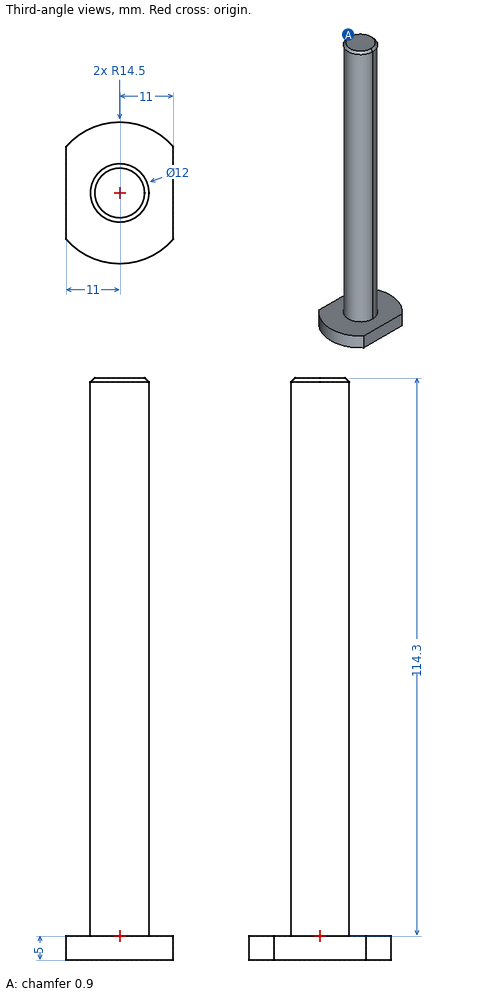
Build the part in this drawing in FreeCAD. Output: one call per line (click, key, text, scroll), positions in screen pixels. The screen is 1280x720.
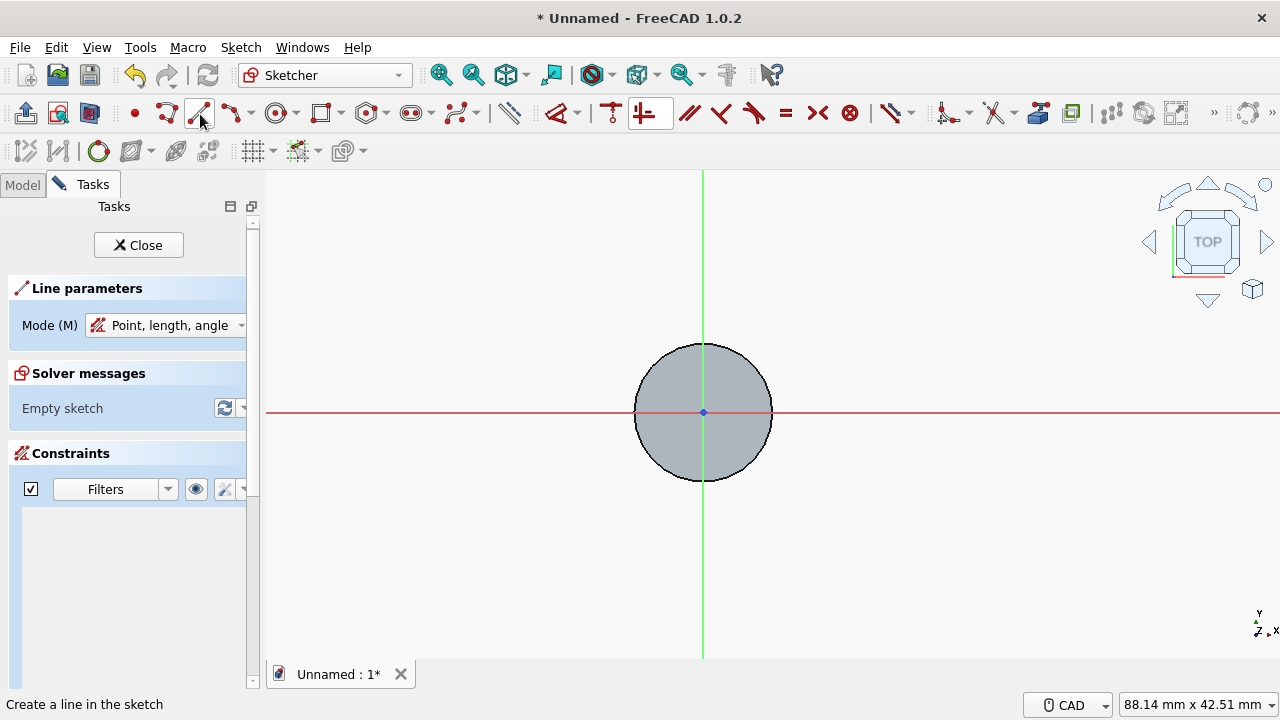
click(577, 521)
click(577, 304)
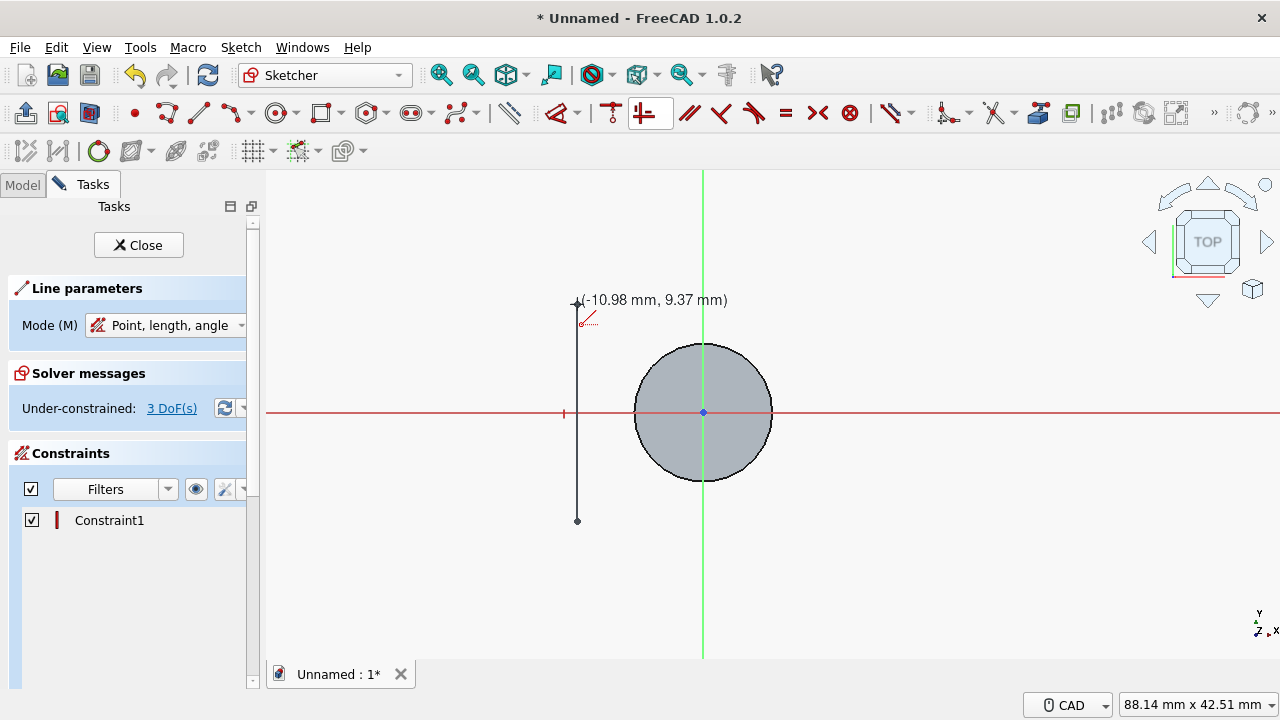
click(830, 304)
click(830, 521)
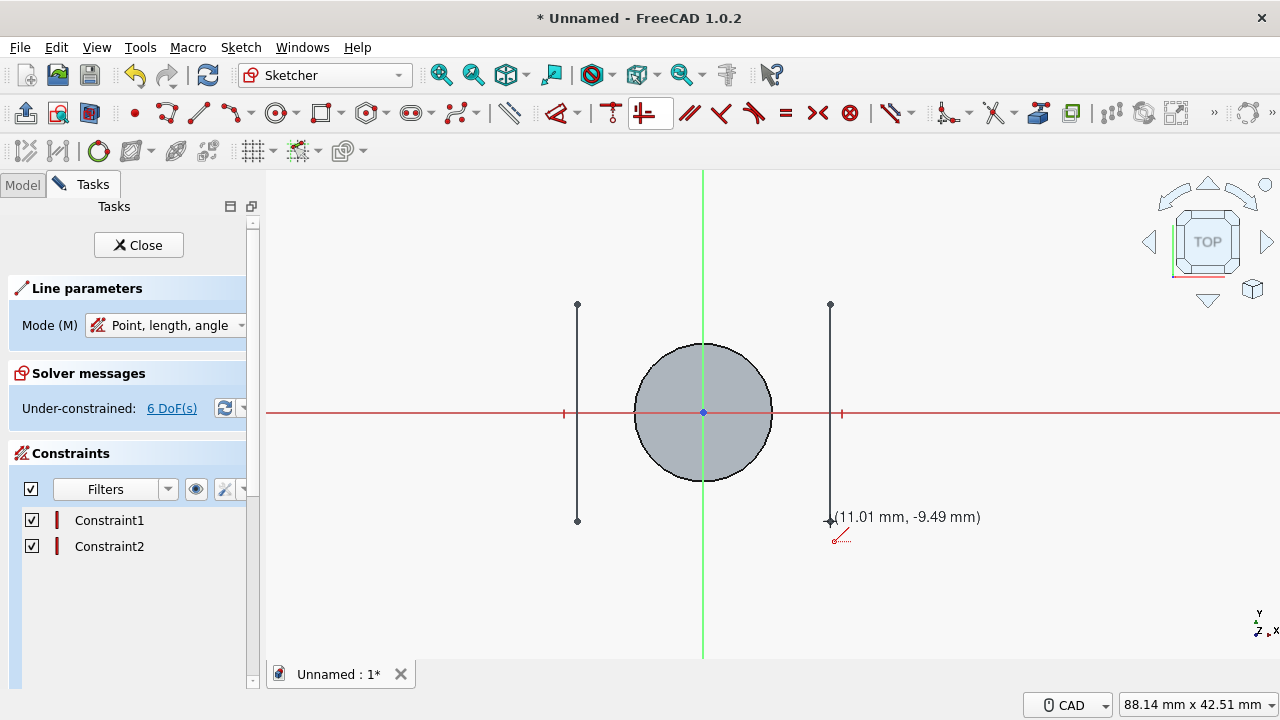
click(232, 114)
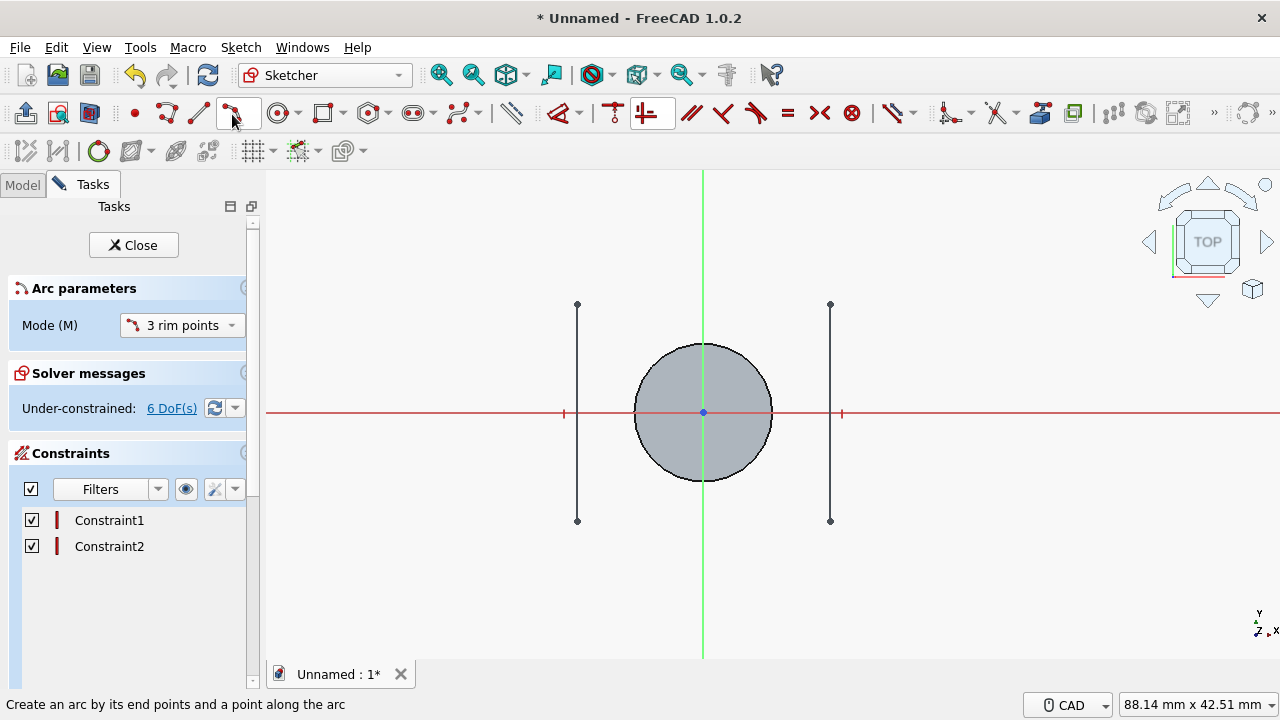
click(577, 305)
click(830, 305)
click(732, 248)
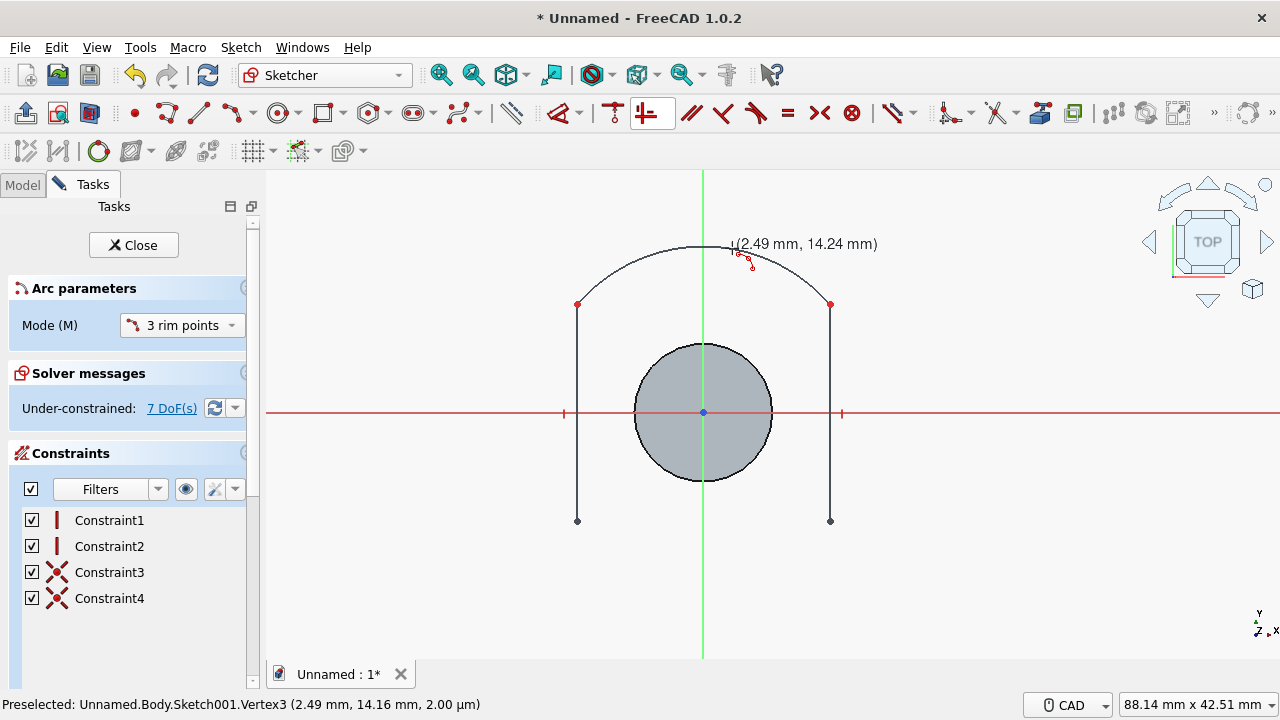
click(830, 522)
click(577, 522)
click(675, 577)
key(Escape)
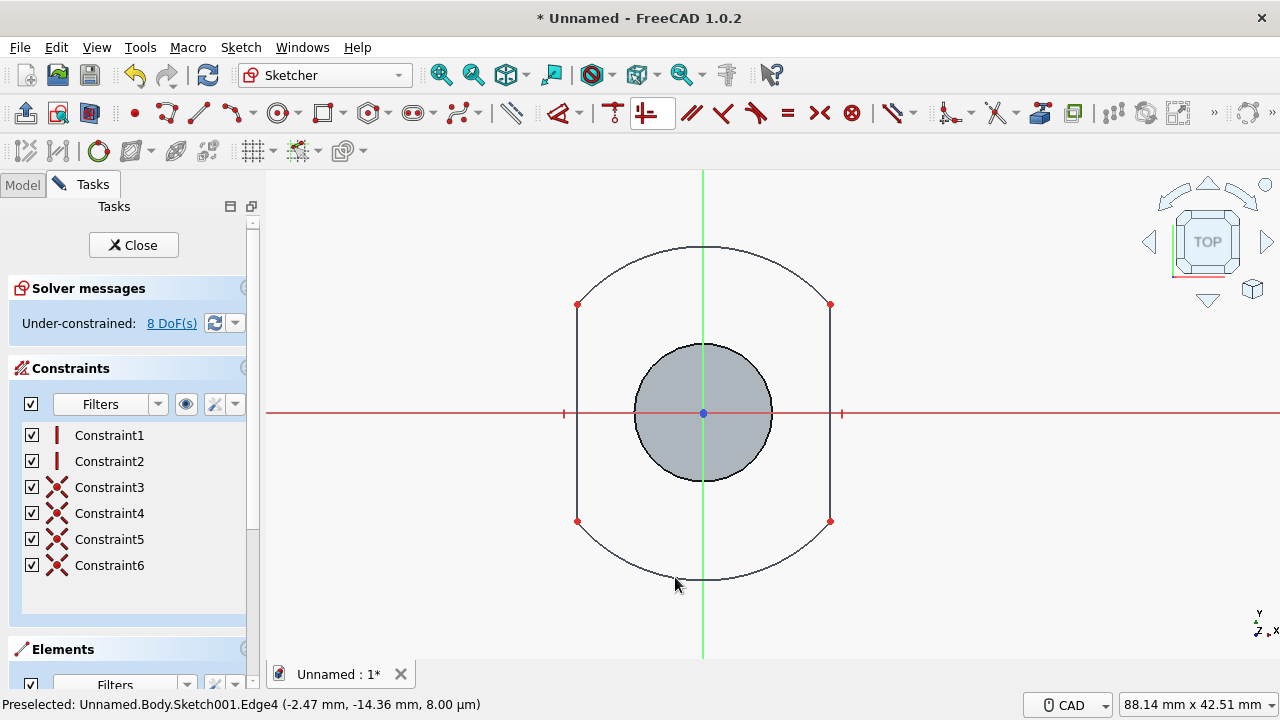
click(760, 256)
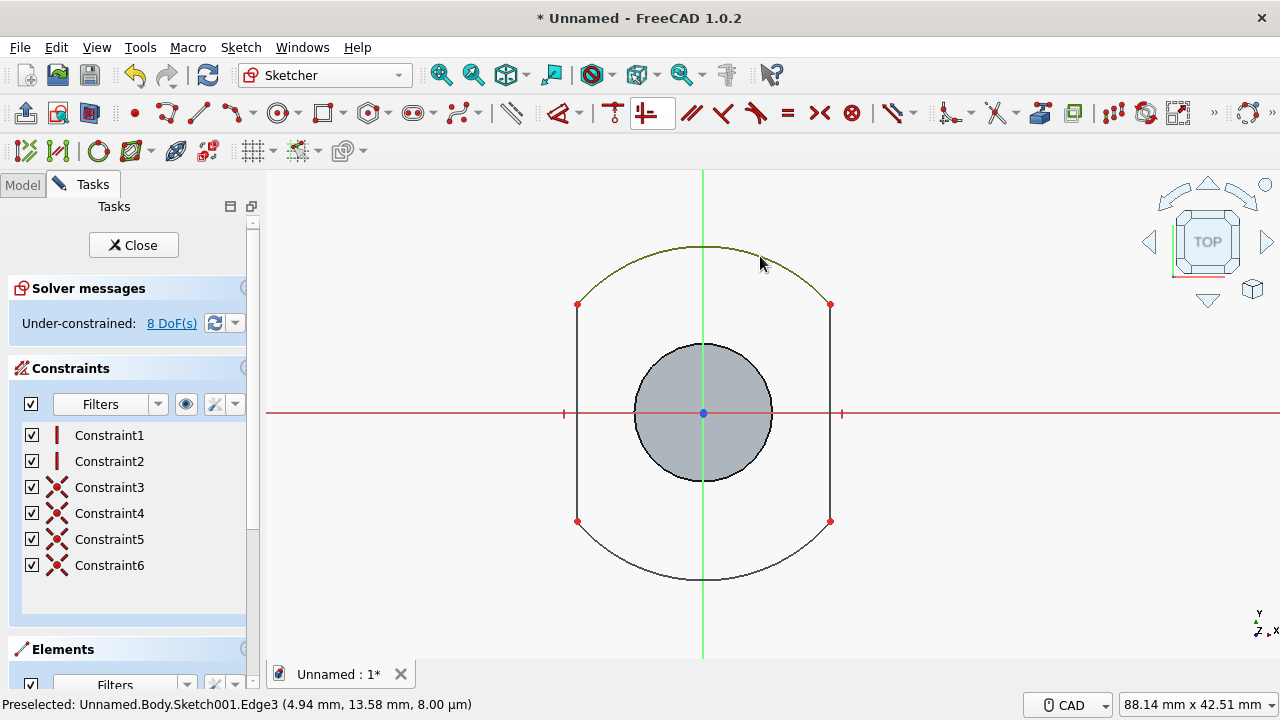
click(647, 571)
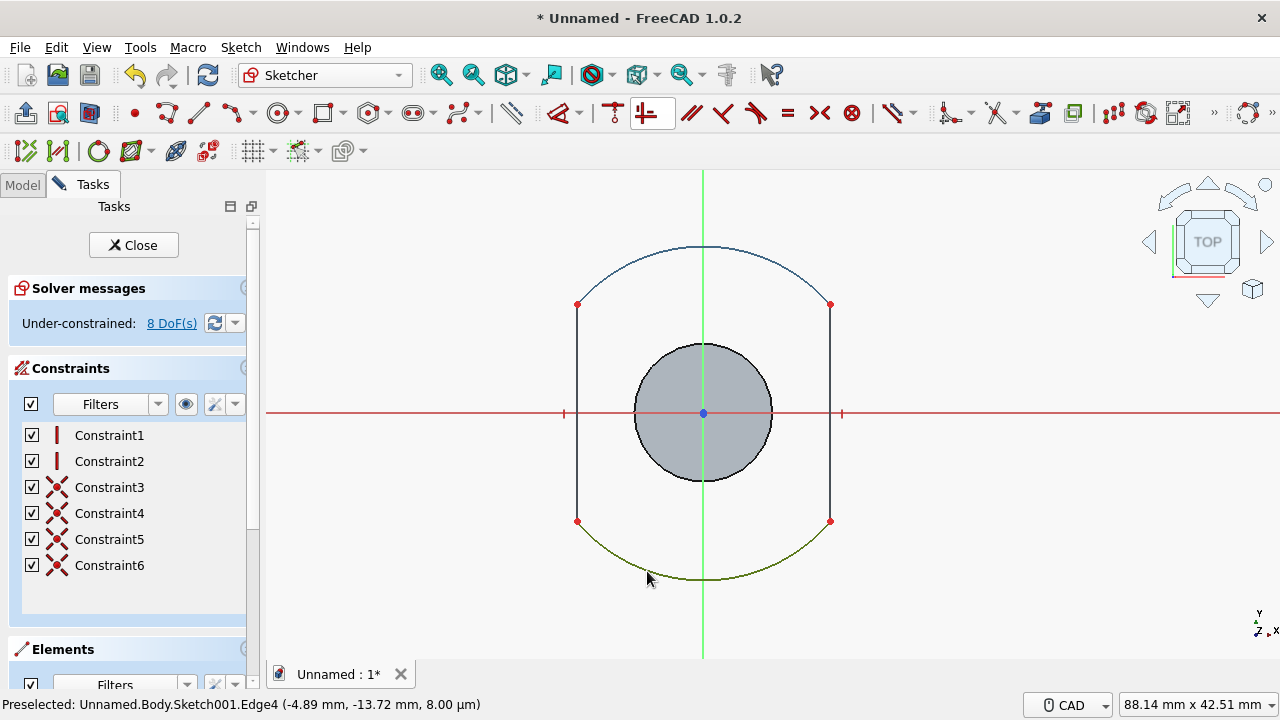
click(614, 114)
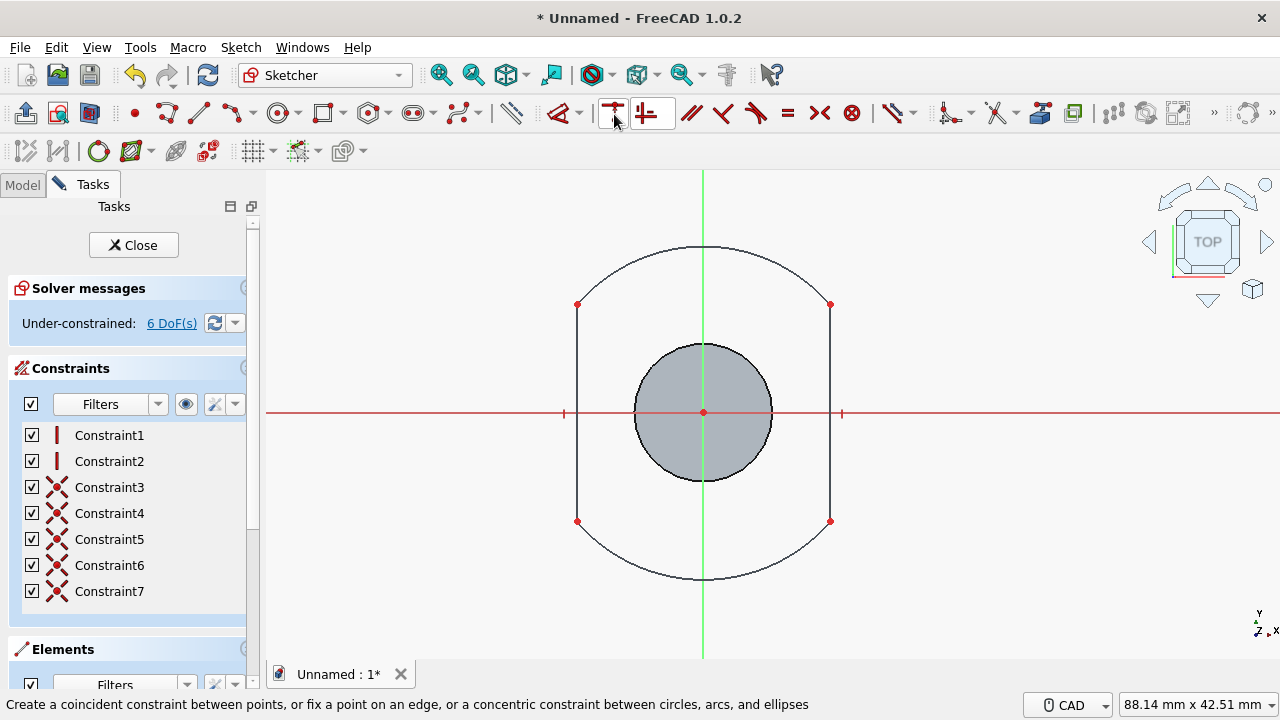
drag(693, 403, 713, 423)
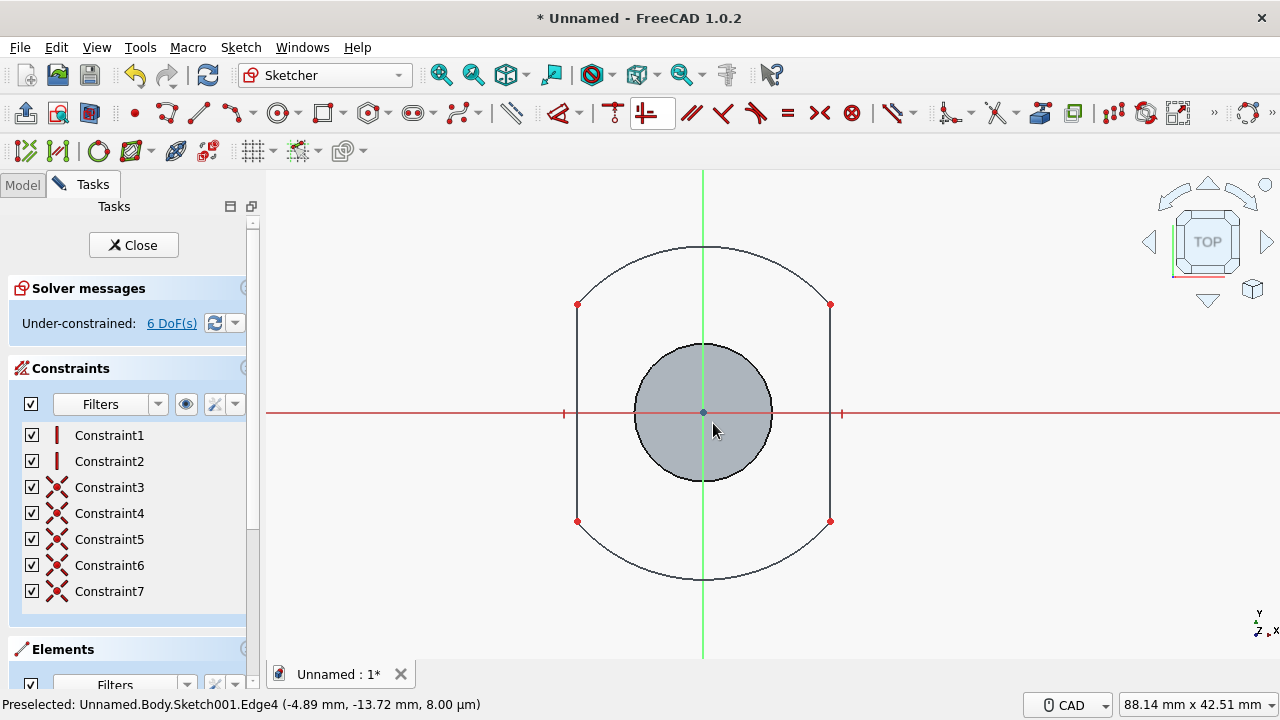
click(614, 114)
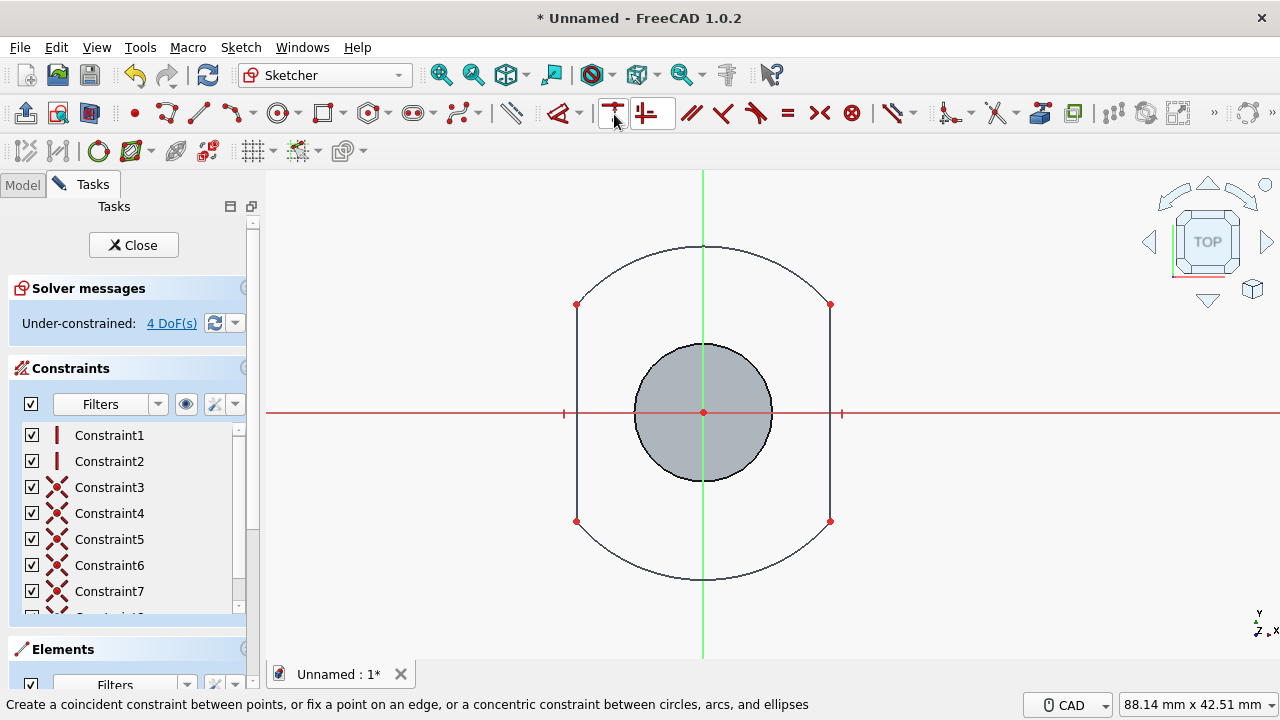
click(760, 256)